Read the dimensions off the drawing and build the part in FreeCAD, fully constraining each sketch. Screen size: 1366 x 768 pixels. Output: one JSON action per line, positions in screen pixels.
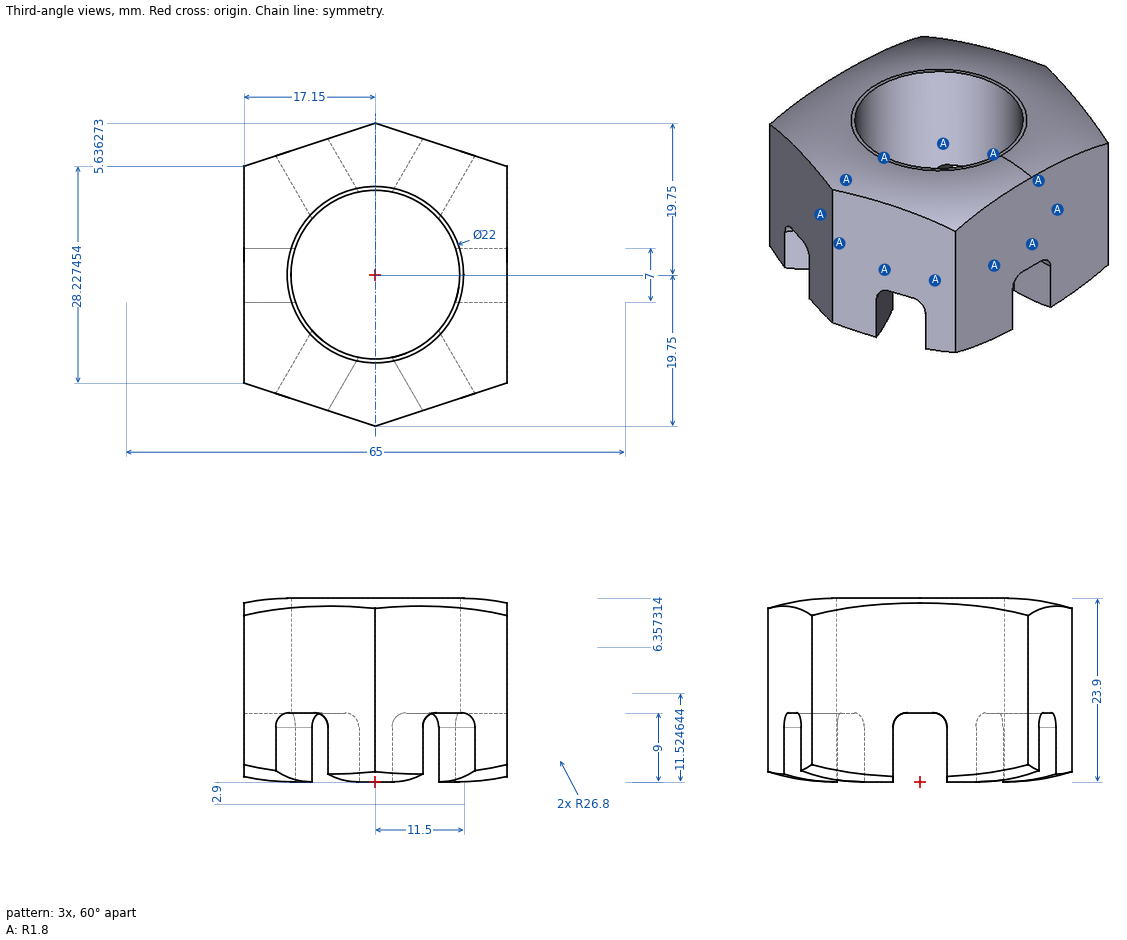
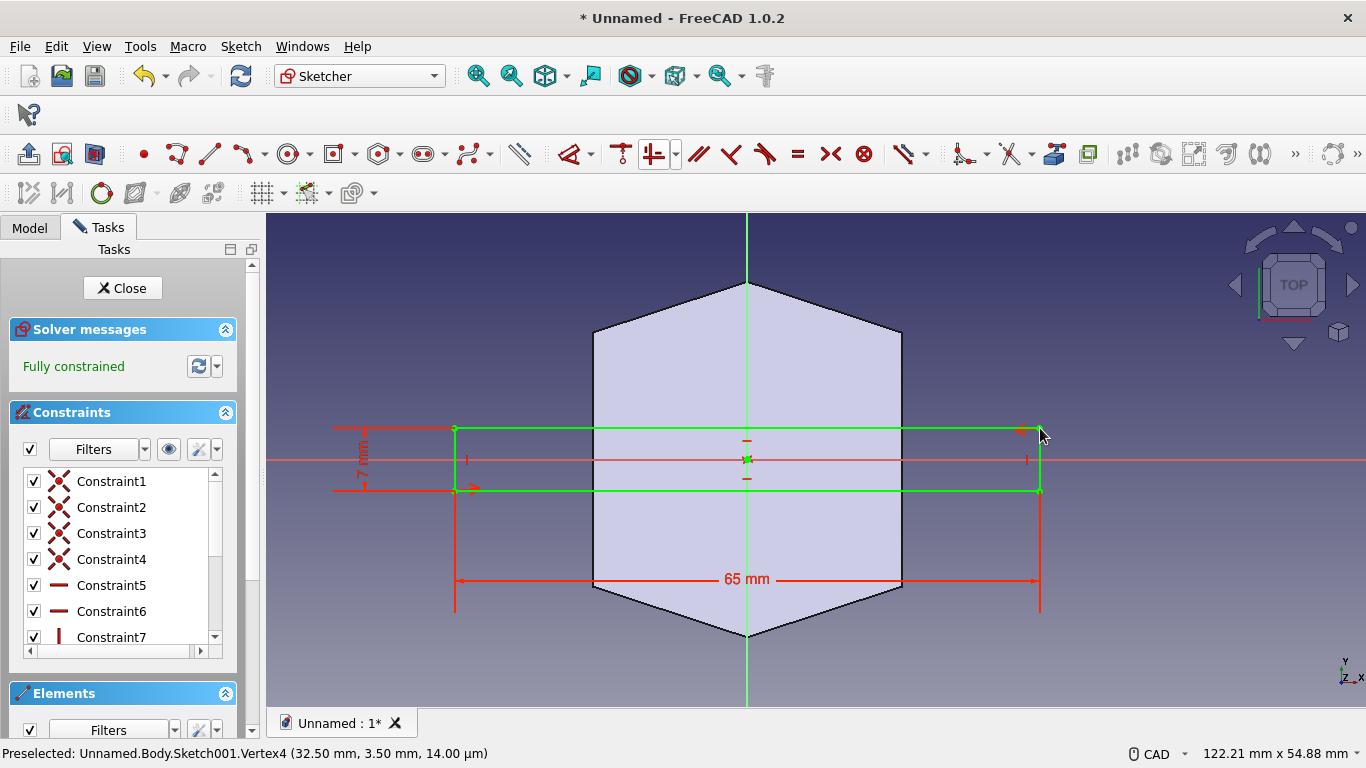
{"action": "left_click", "coordinate": [123, 288]}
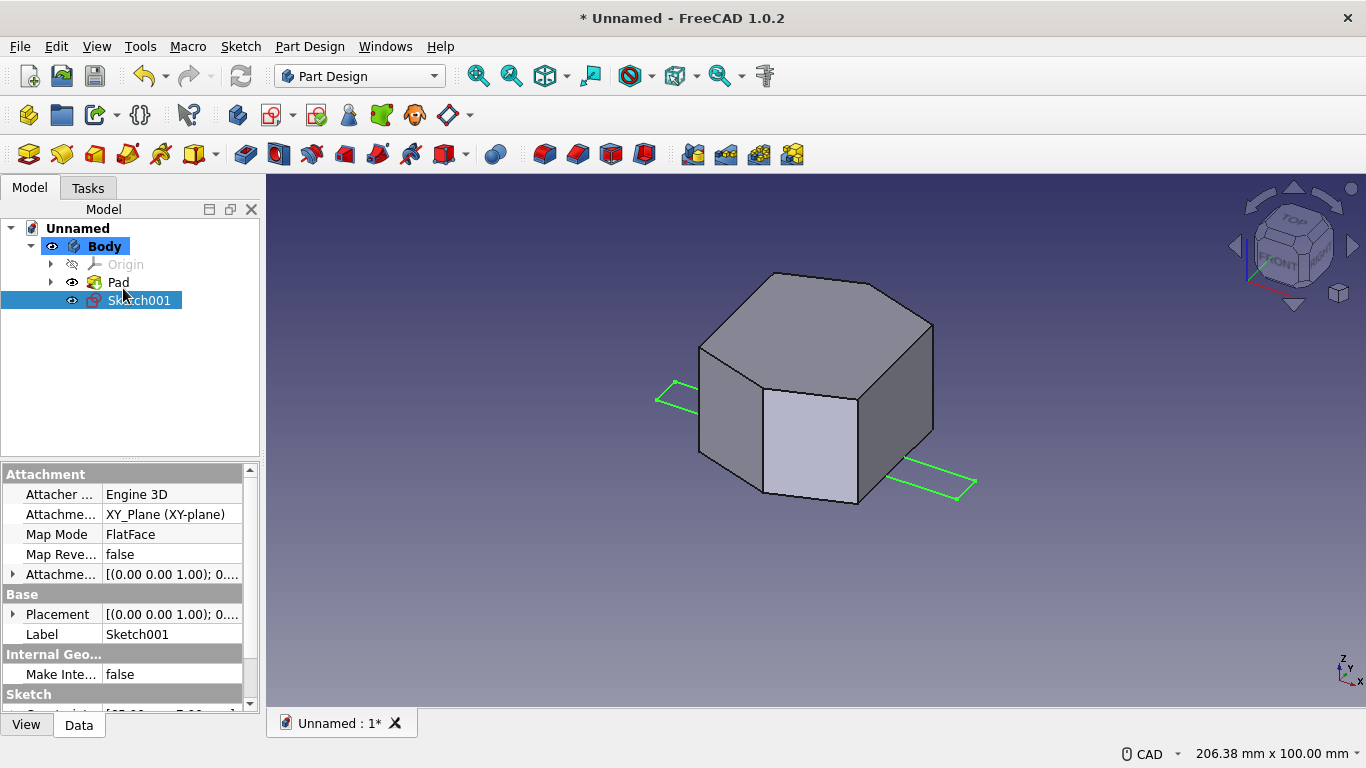
{"action": "left_click", "coordinate": [246, 154]}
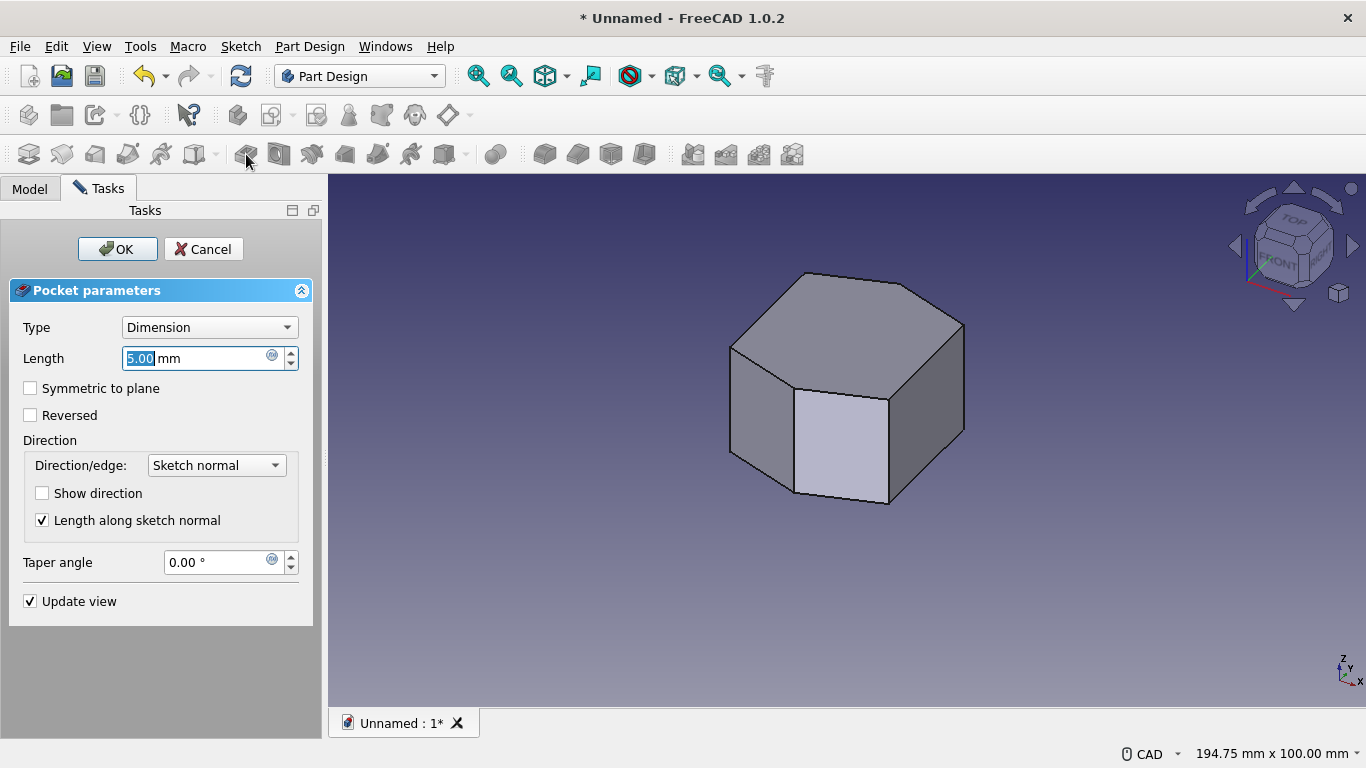
{"action": "type", "text": "9"}
{"action": "key", "text": "Tab"}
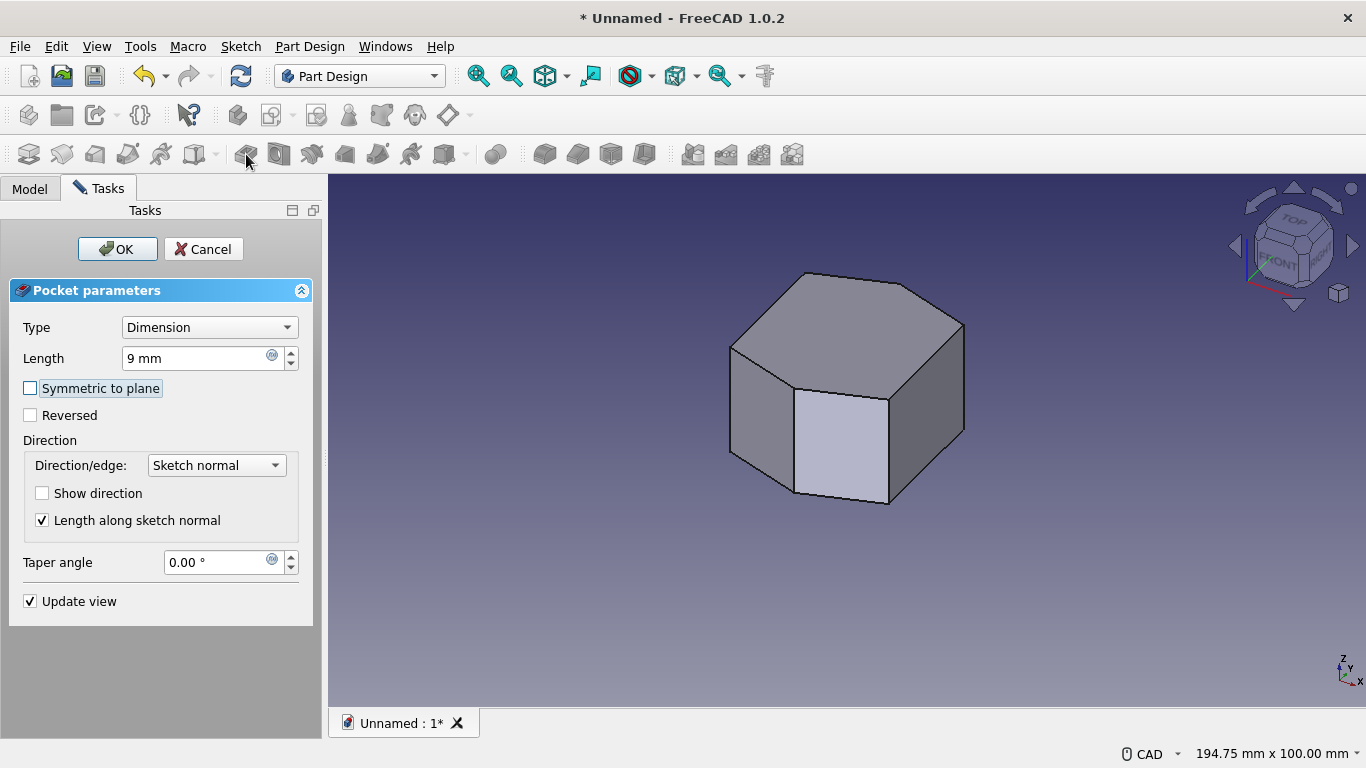
{"action": "left_click", "coordinate": [31, 415]}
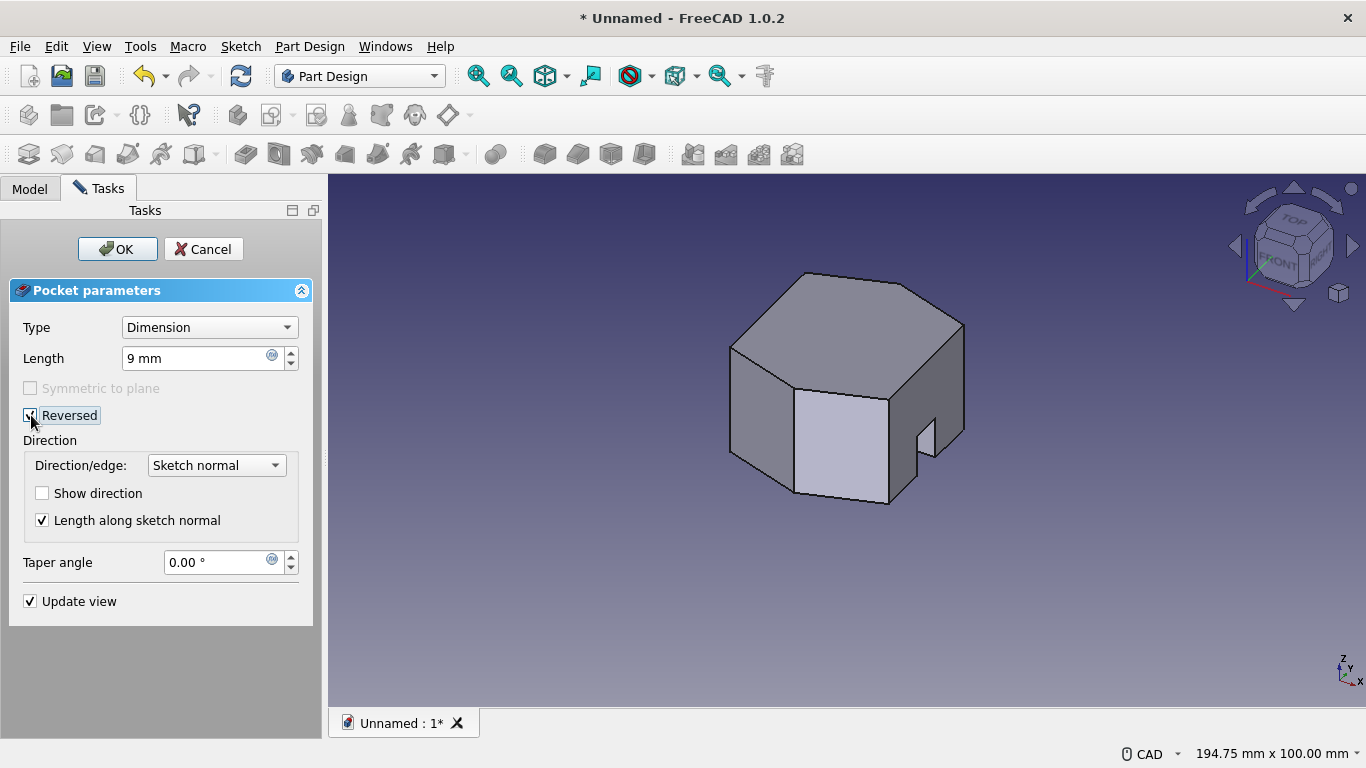
{"action": "left_click", "coordinate": [118, 249]}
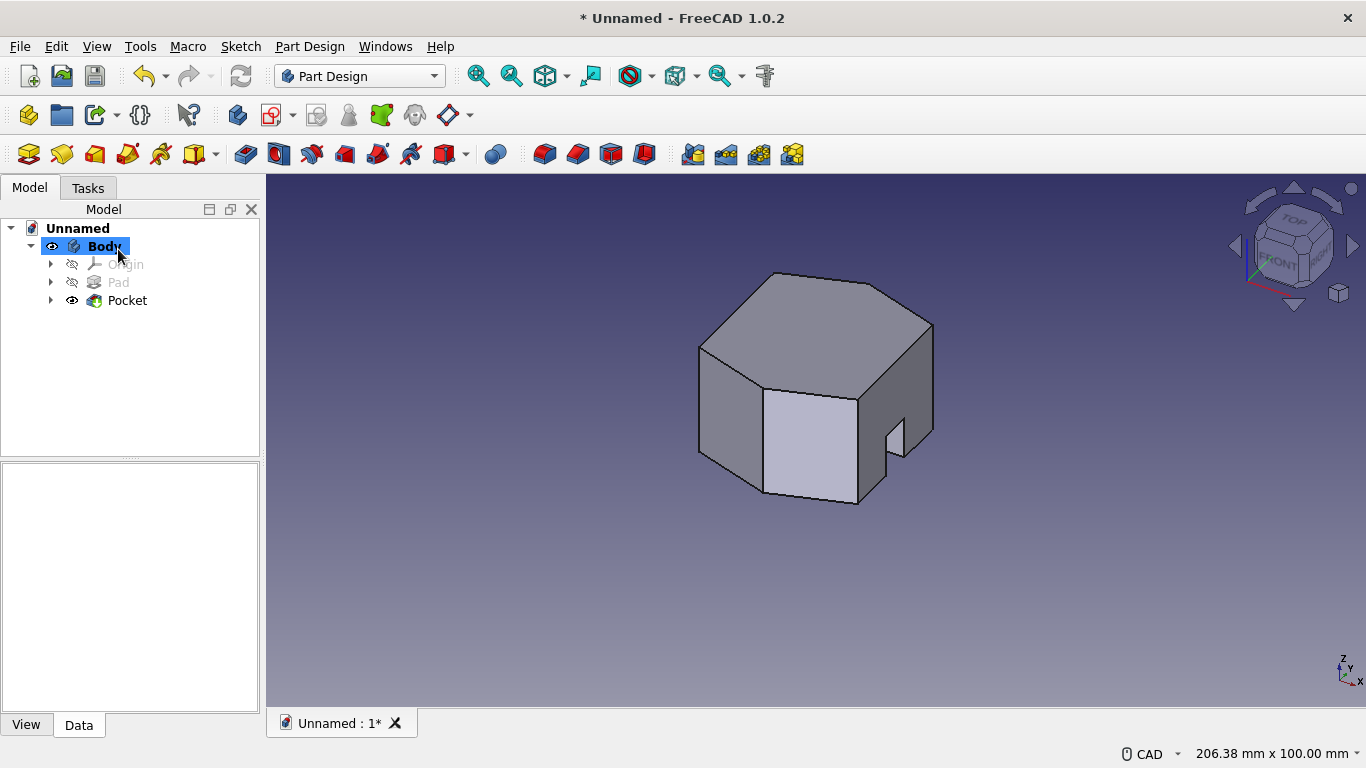
{"action": "left_click", "coordinate": [117, 300]}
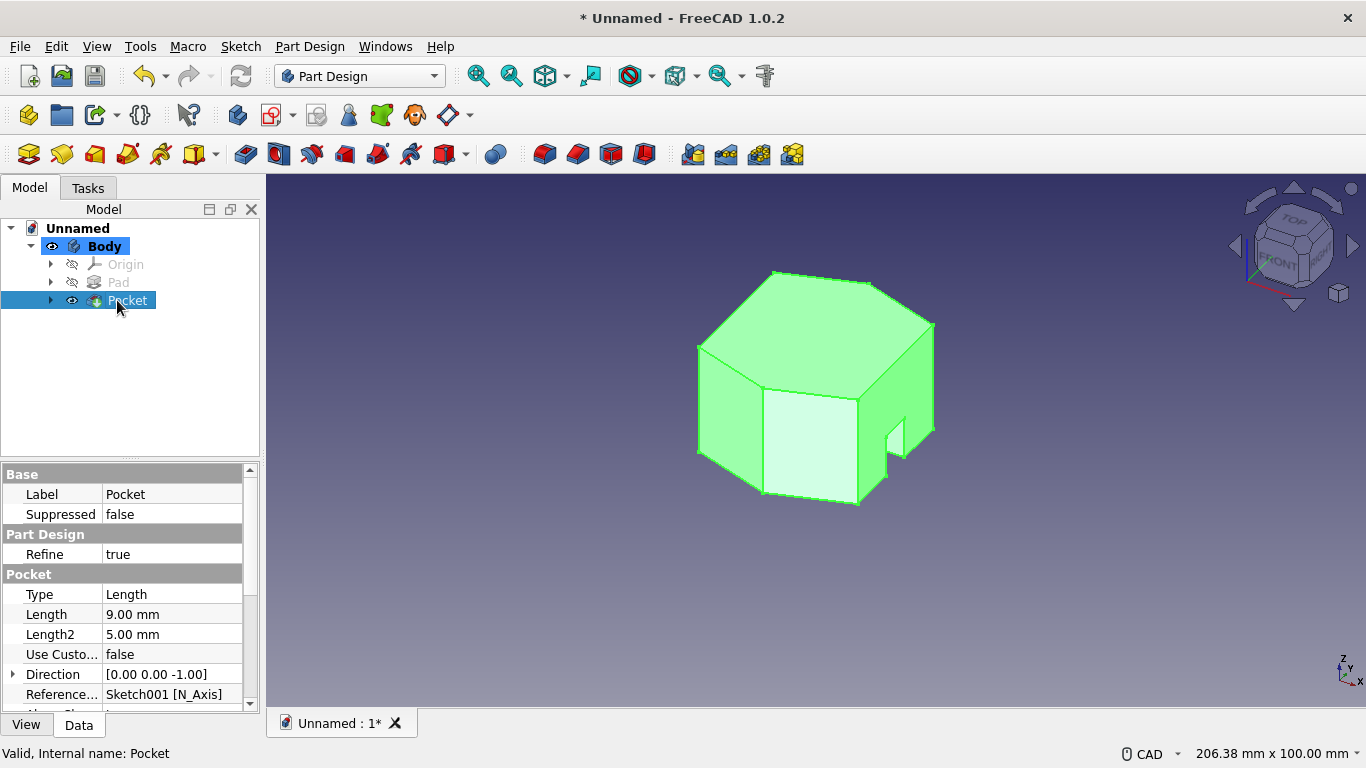
{"action": "left_click", "coordinate": [759, 154]}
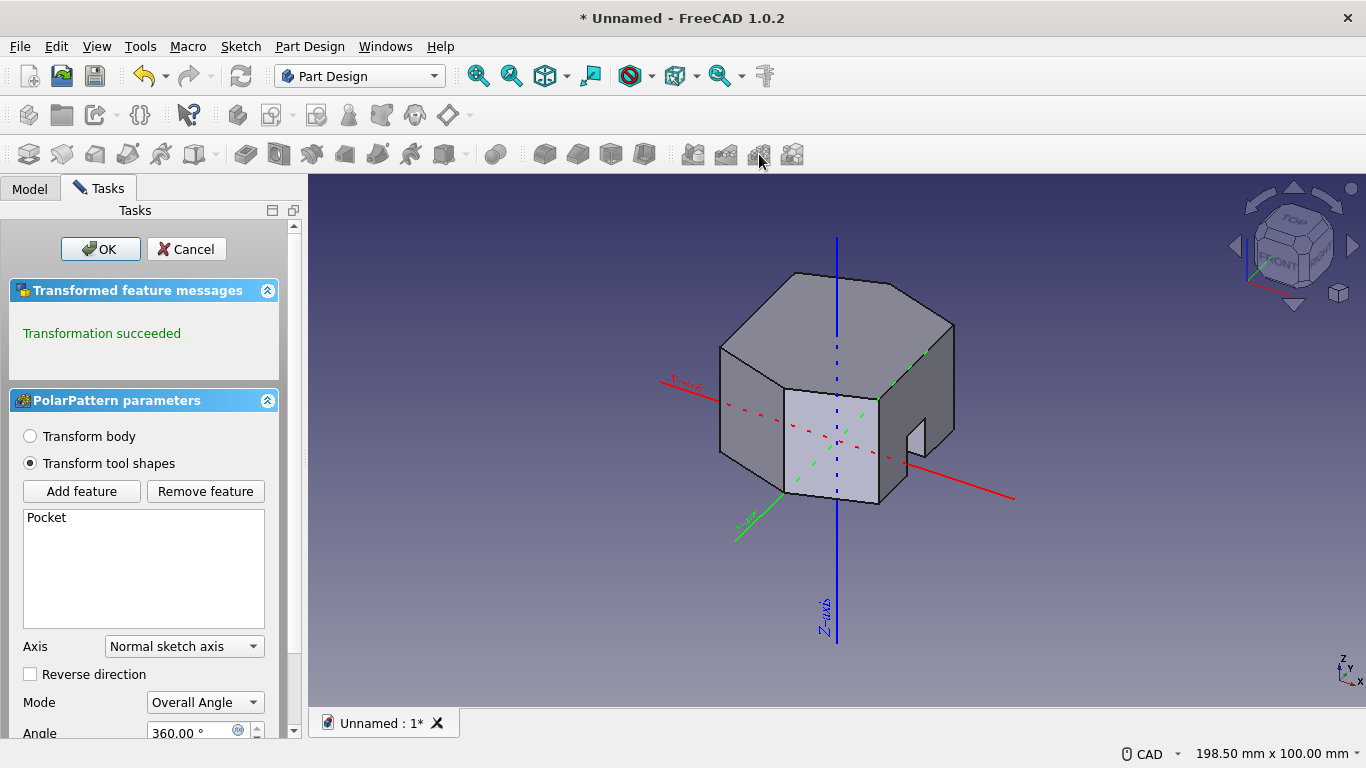
{"action": "left_click", "coordinate": [185, 646]}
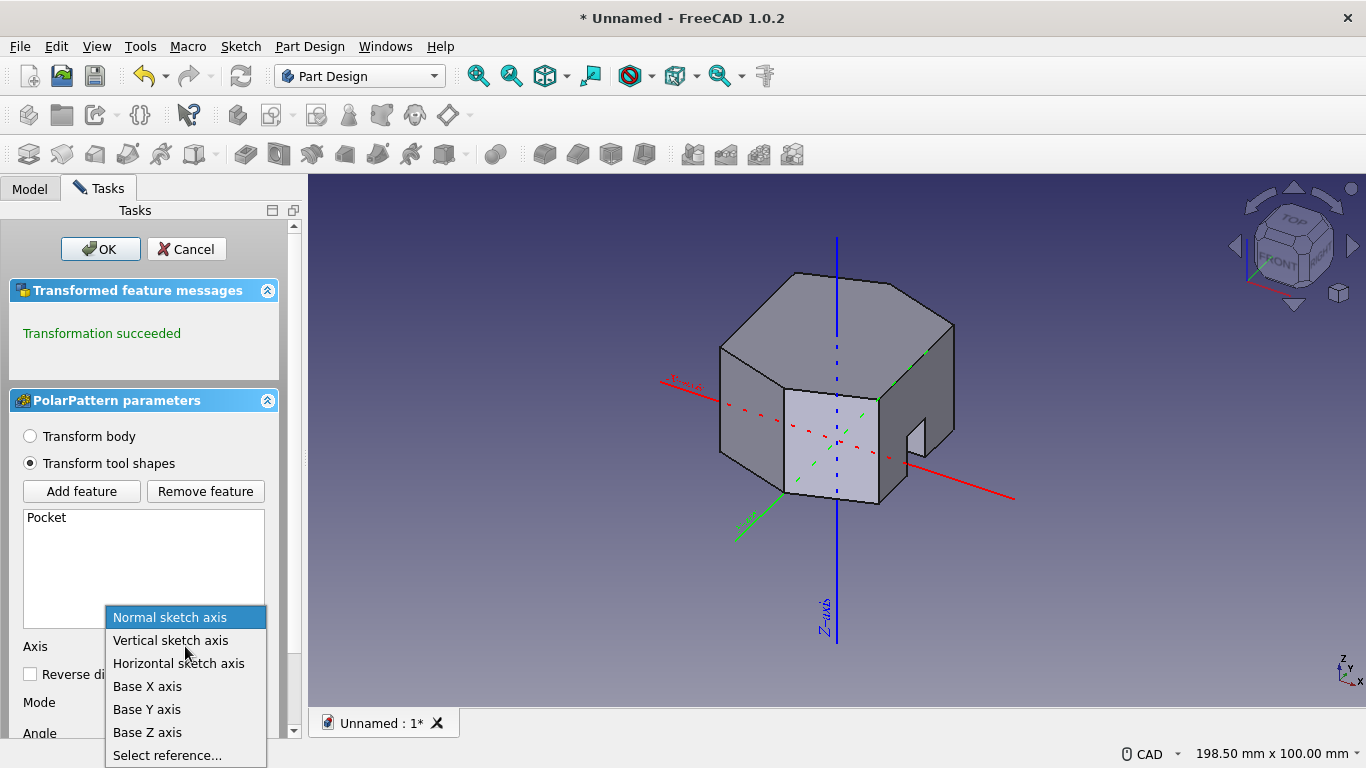
{"action": "left_click", "coordinate": [184, 732]}